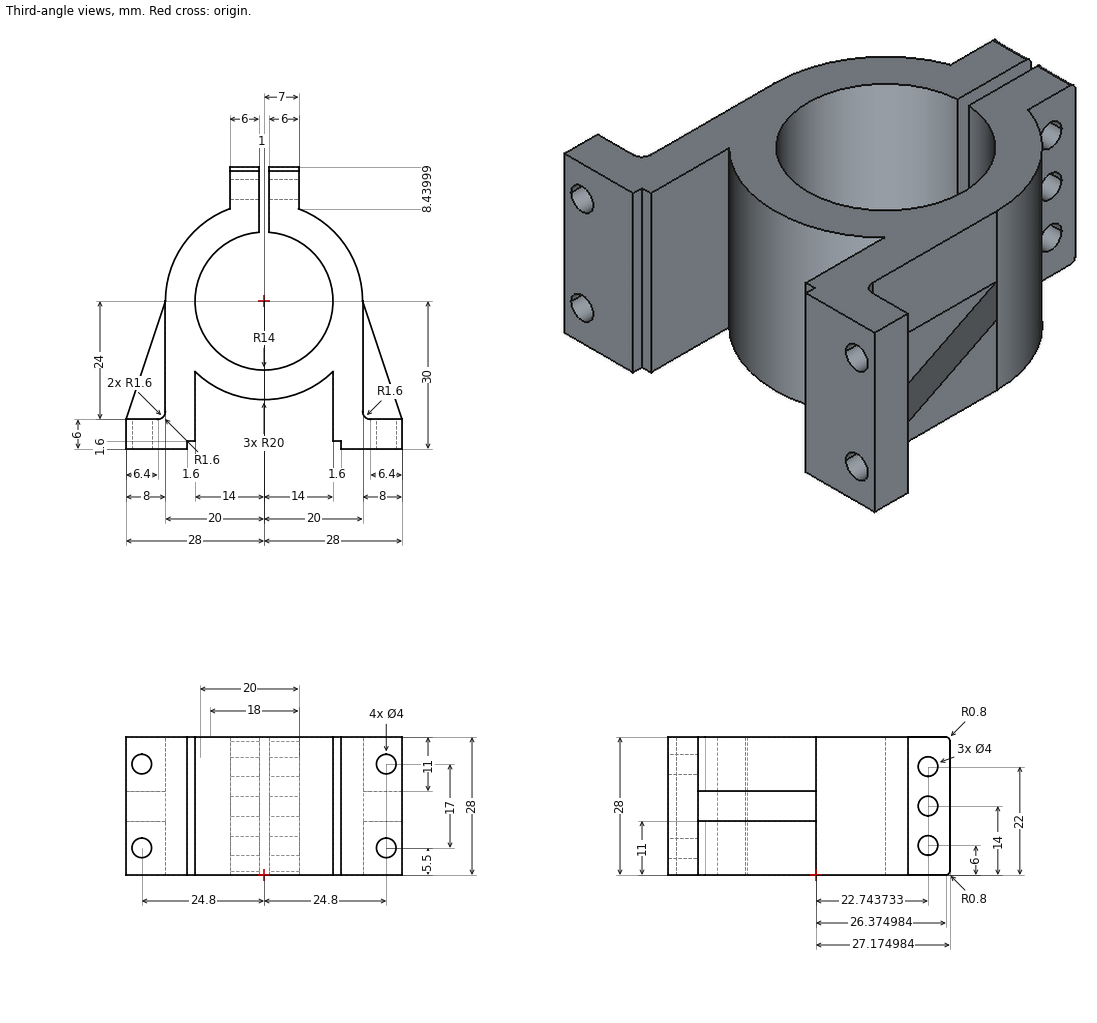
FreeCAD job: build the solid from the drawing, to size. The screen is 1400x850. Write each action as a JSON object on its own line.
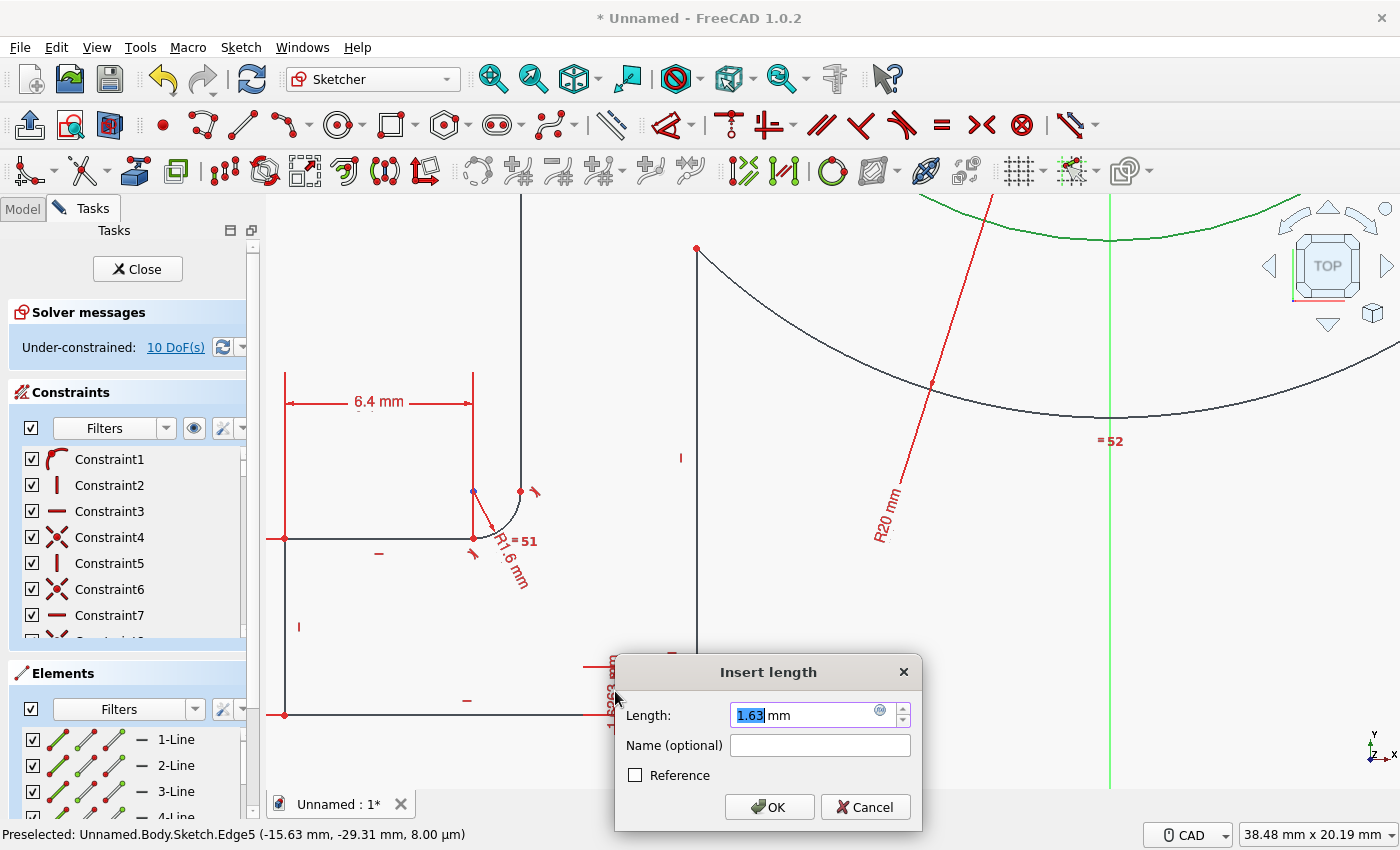
{"action": "type", "text": "1.6"}
{"action": "key", "text": "Return"}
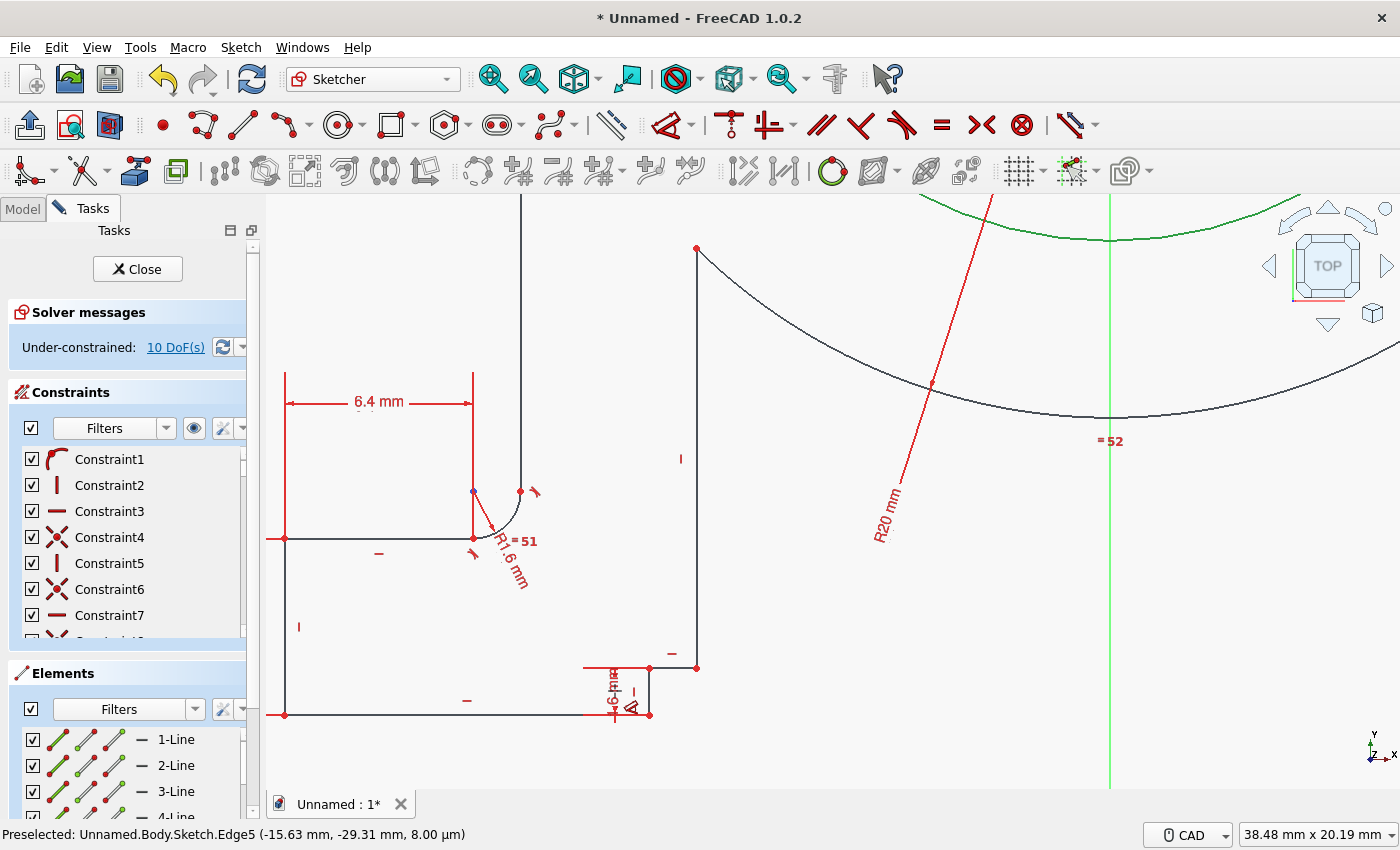
{"action": "left_click", "coordinate": [664, 668]}
{"action": "left_click", "coordinate": [689, 702]}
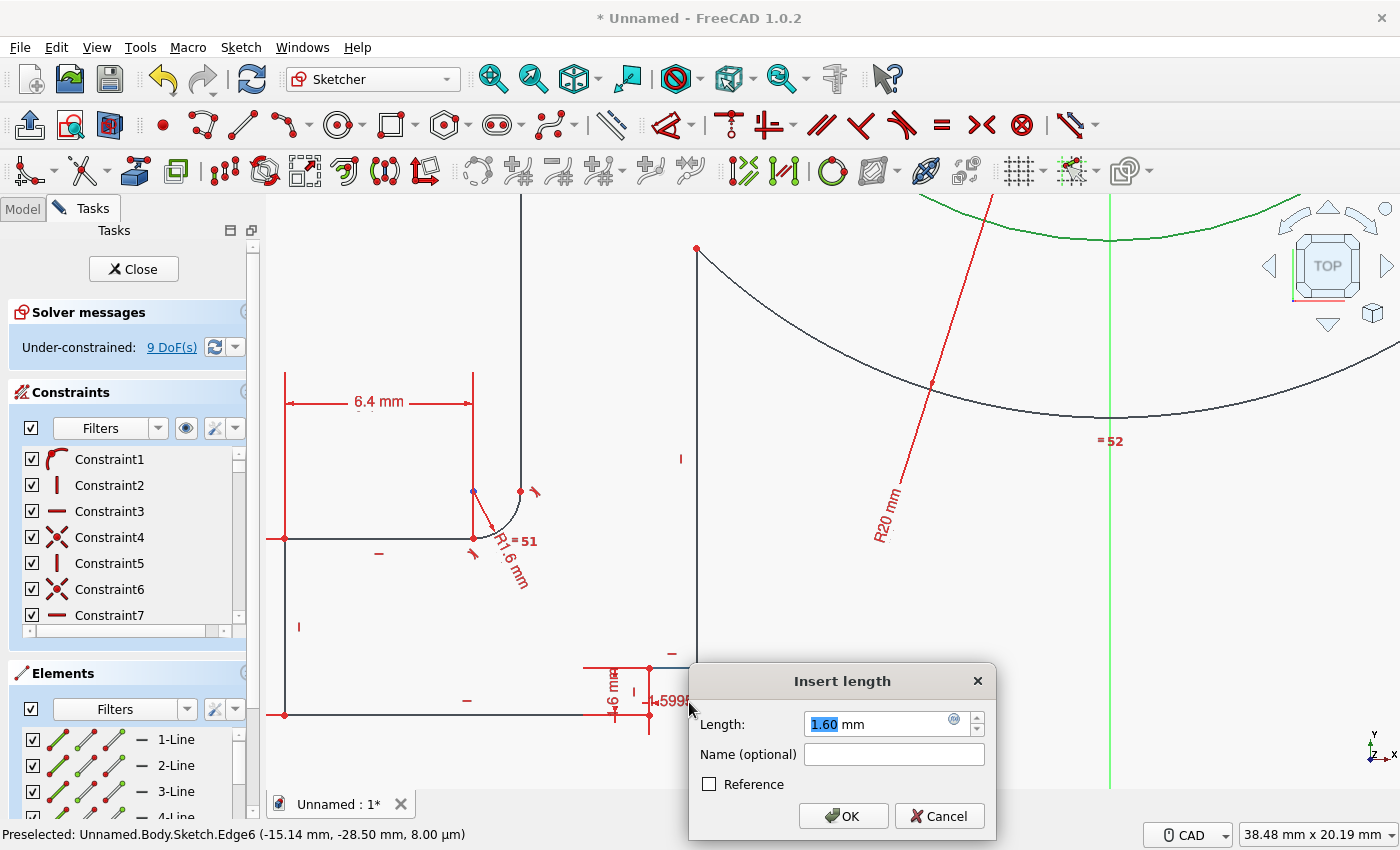
{"action": "type", "text": "1.6"}
{"action": "key", "text": "Return"}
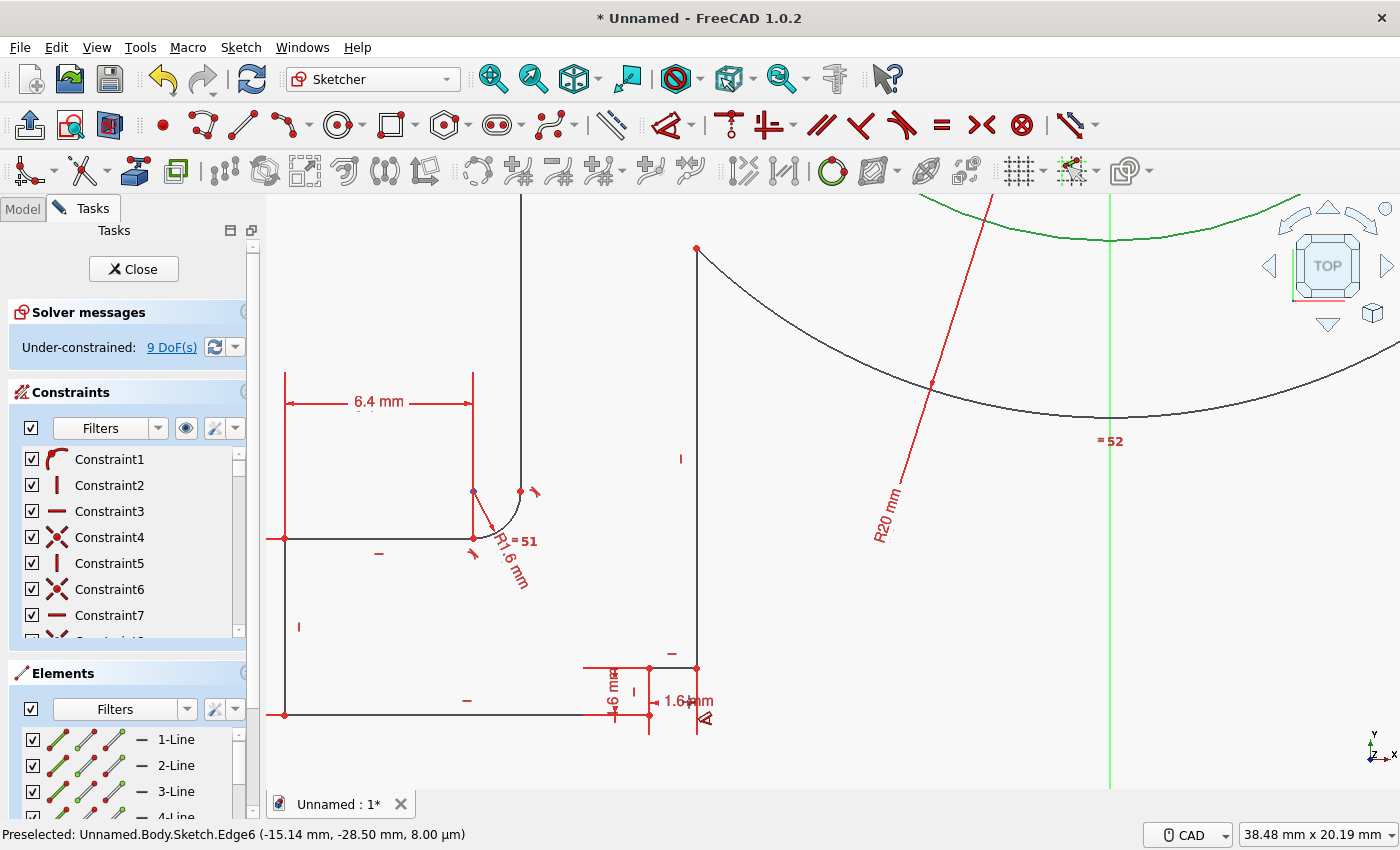
{"action": "scroll", "coordinate": [651, 695], "scroll_direction": "down", "scroll_amount": 7}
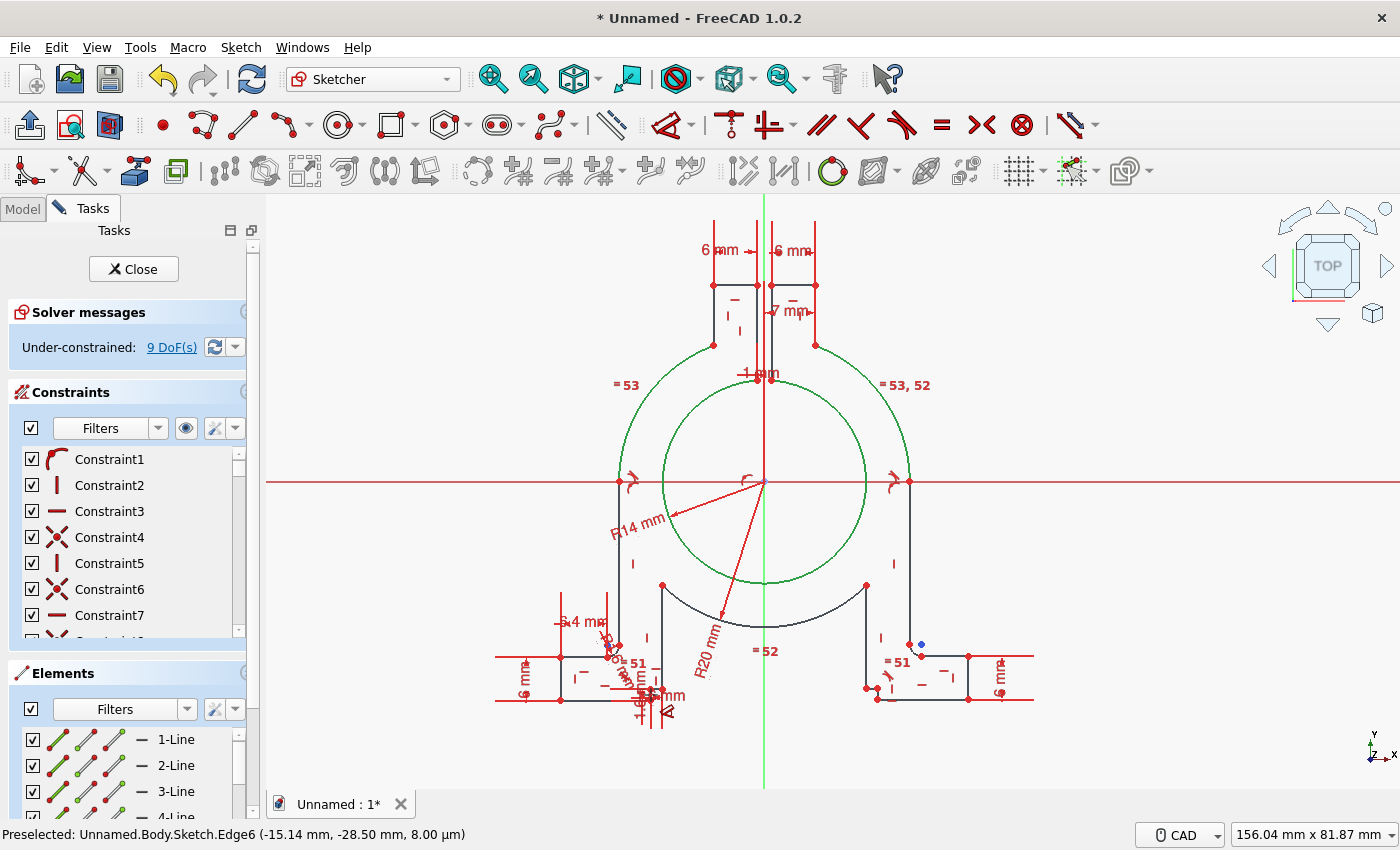
{"action": "scroll", "coordinate": [870, 689], "scroll_direction": "up", "scroll_amount": 7}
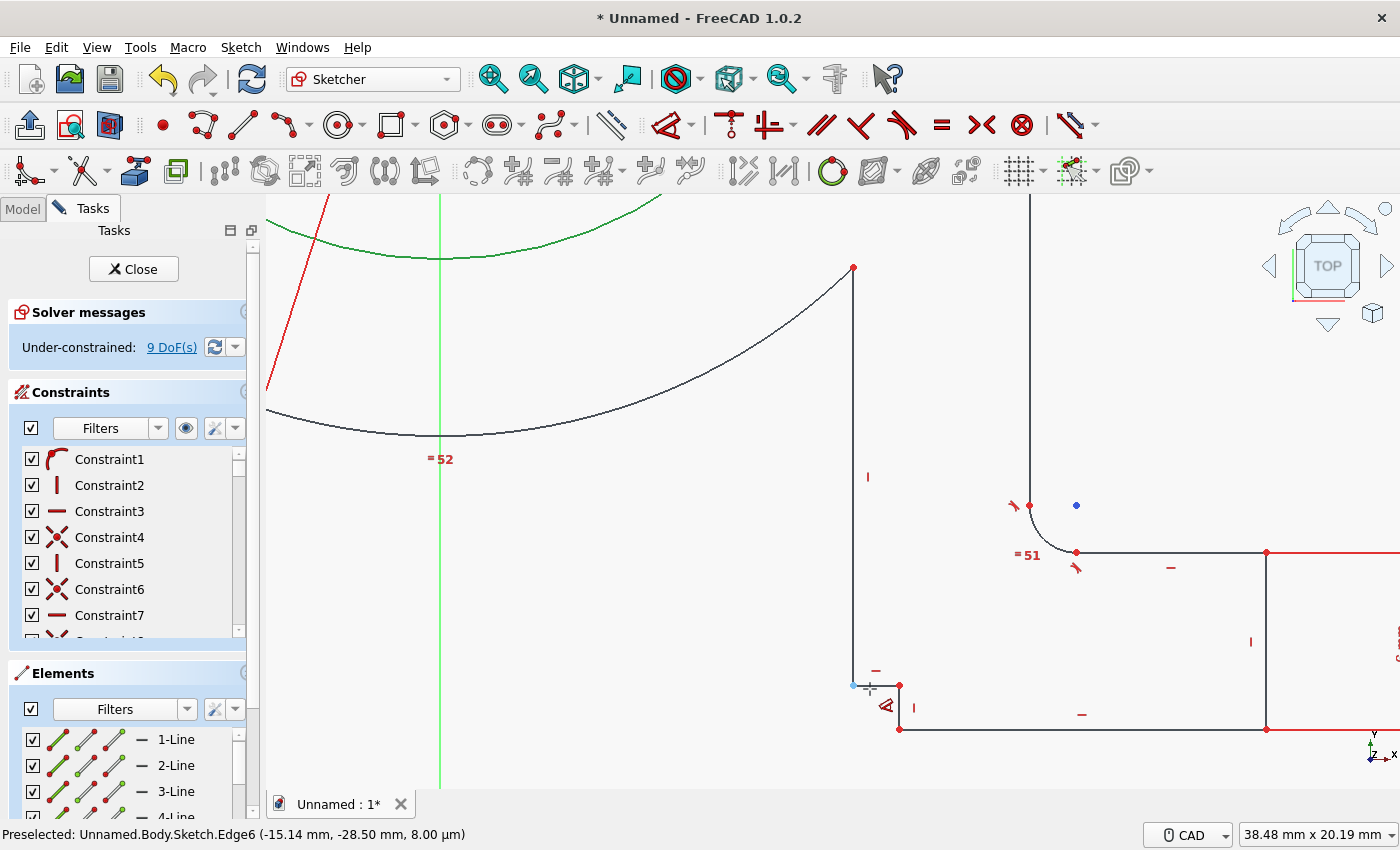
{"action": "left_click", "coordinate": [867, 686]}
{"action": "left_click", "coordinate": [876, 720]}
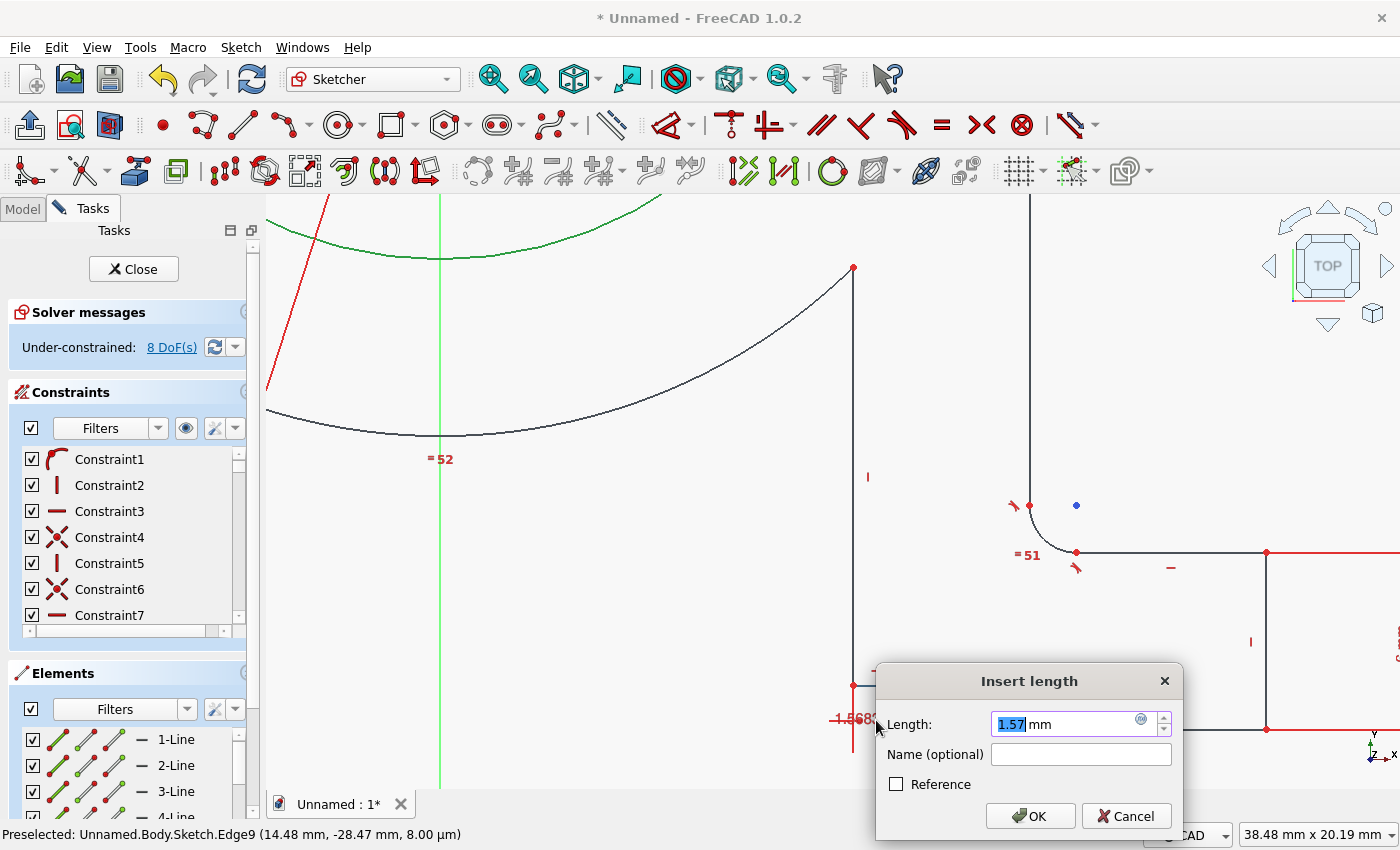
{"action": "type", "text": "1.6"}
{"action": "key", "text": "Return"}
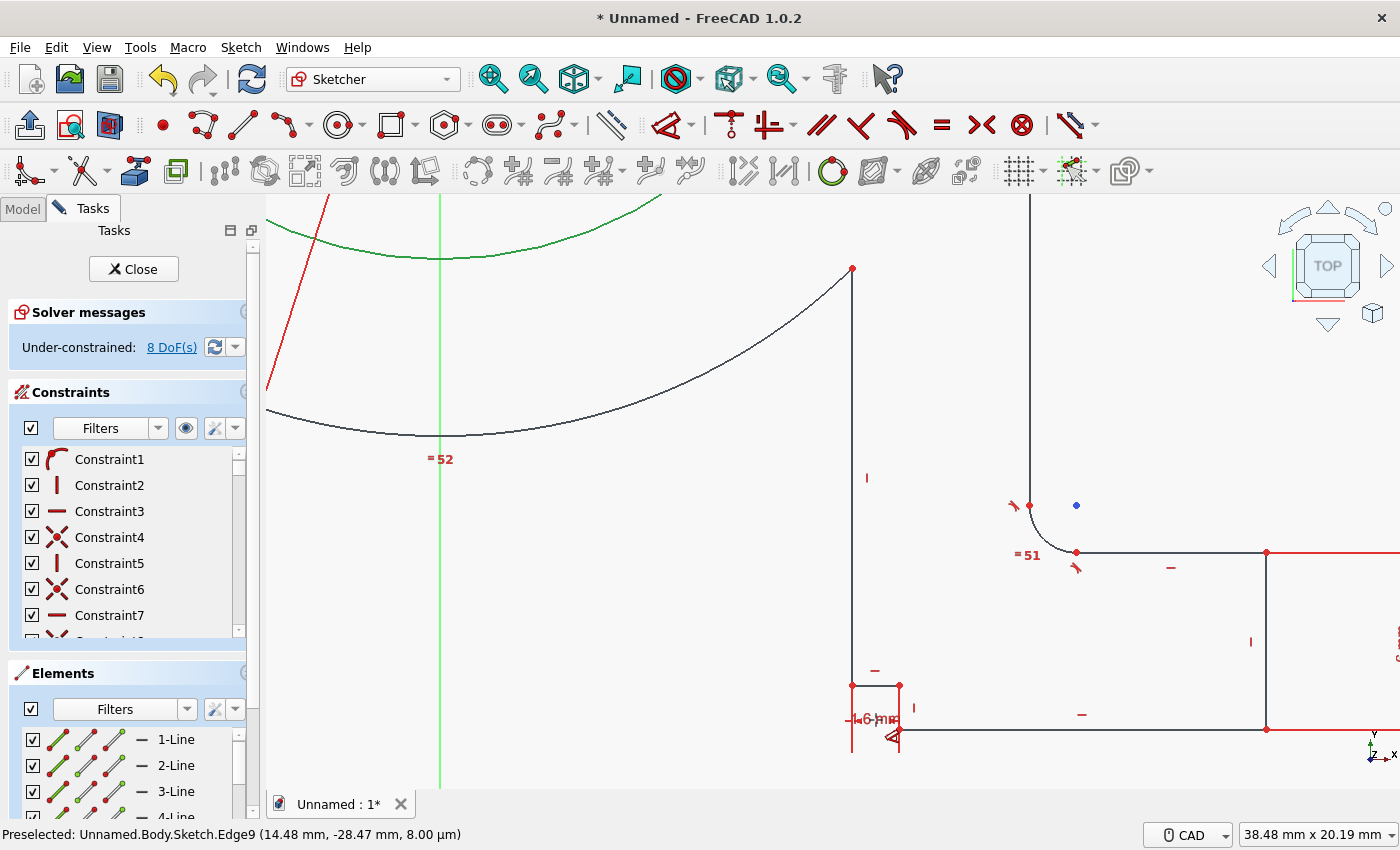
{"action": "left_click", "coordinate": [899, 699]}
{"action": "left_click", "coordinate": [933, 698]}